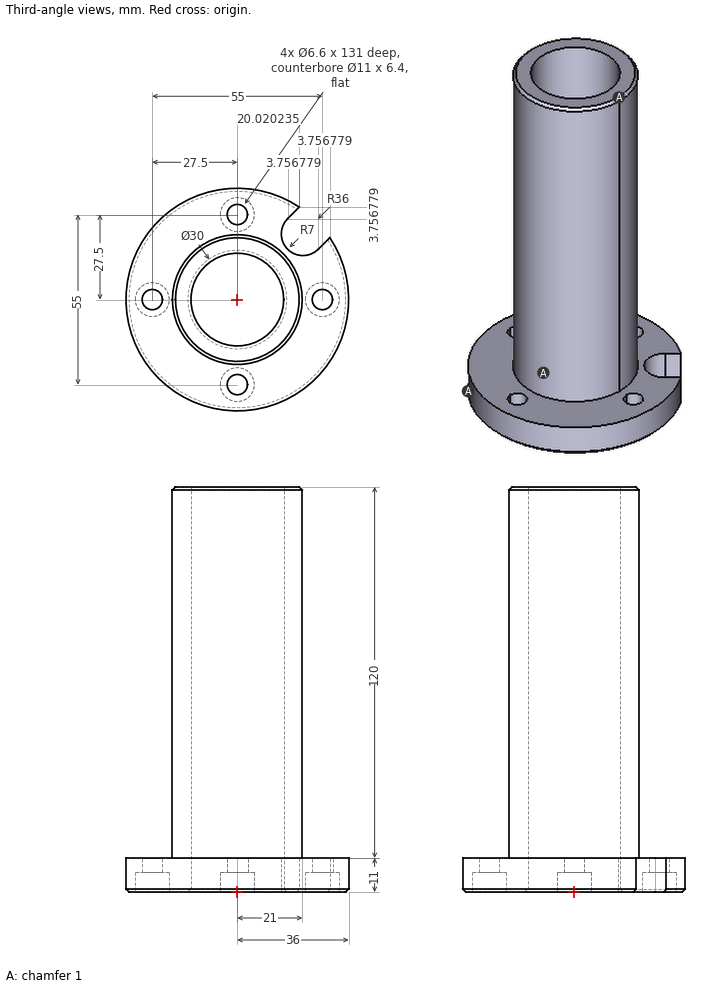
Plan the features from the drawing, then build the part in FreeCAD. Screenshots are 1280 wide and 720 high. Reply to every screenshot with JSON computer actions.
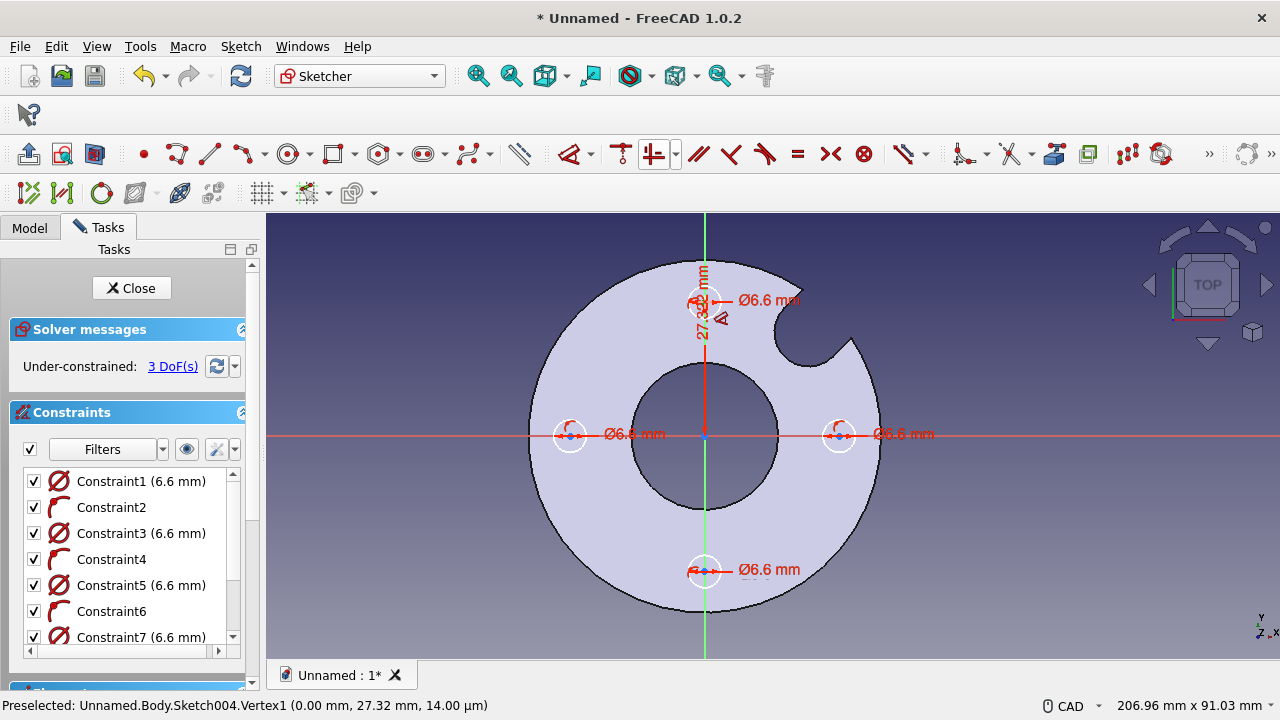
{"action": "left_click", "coordinate": [705, 572]}
{"action": "left_click", "coordinate": [739, 375]}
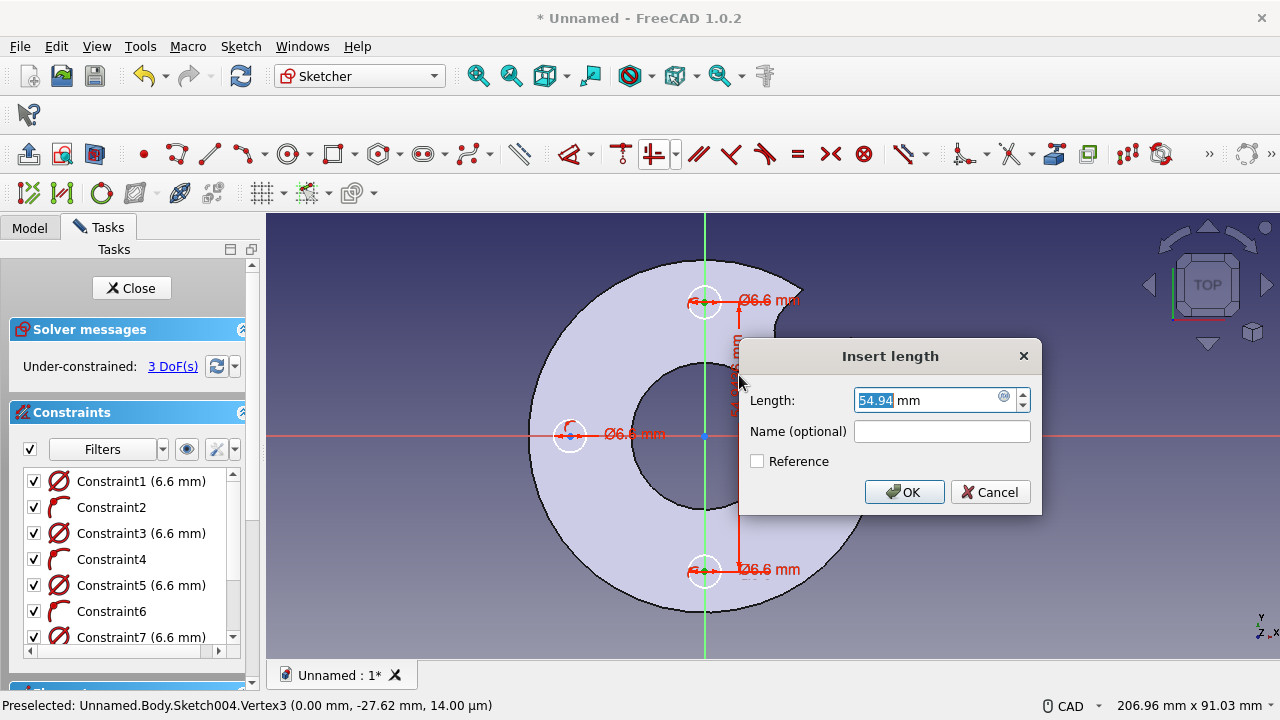
{"action": "type", "text": "55"}
{"action": "key", "text": "Return"}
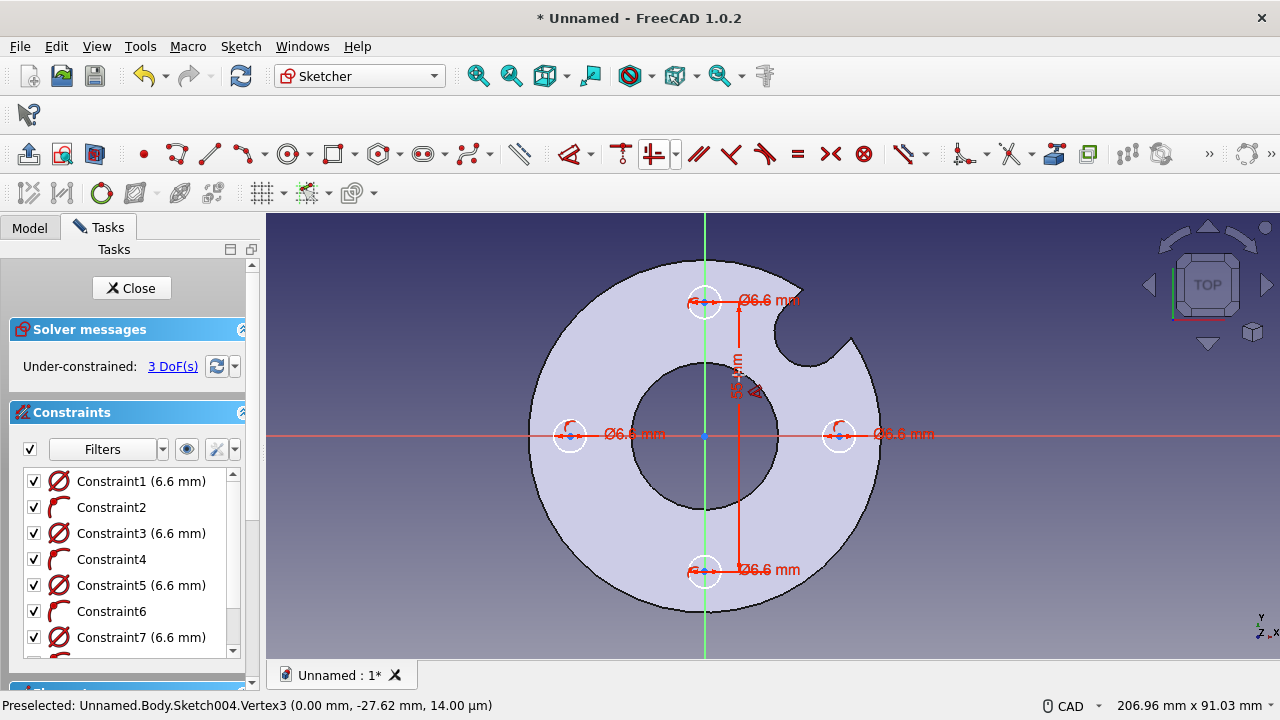
{"action": "left_click", "coordinate": [570, 436]}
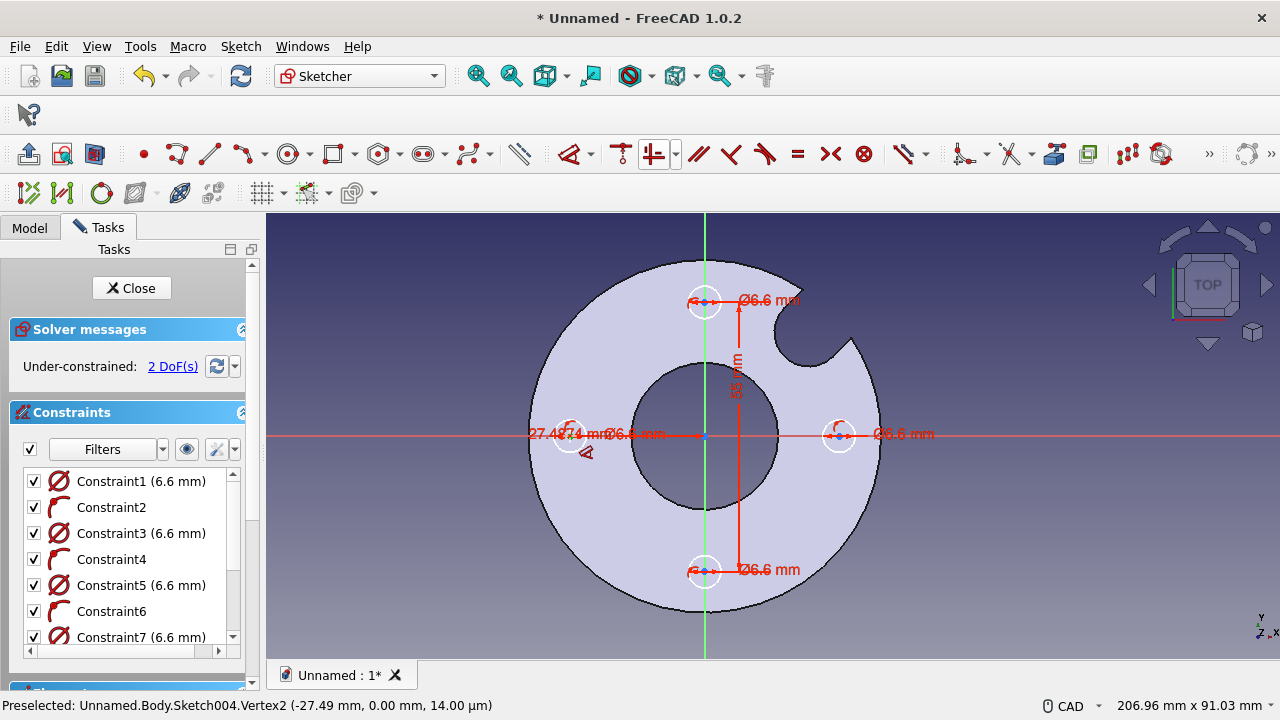
{"action": "left_click", "coordinate": [839, 436]}
{"action": "left_click", "coordinate": [643, 470]}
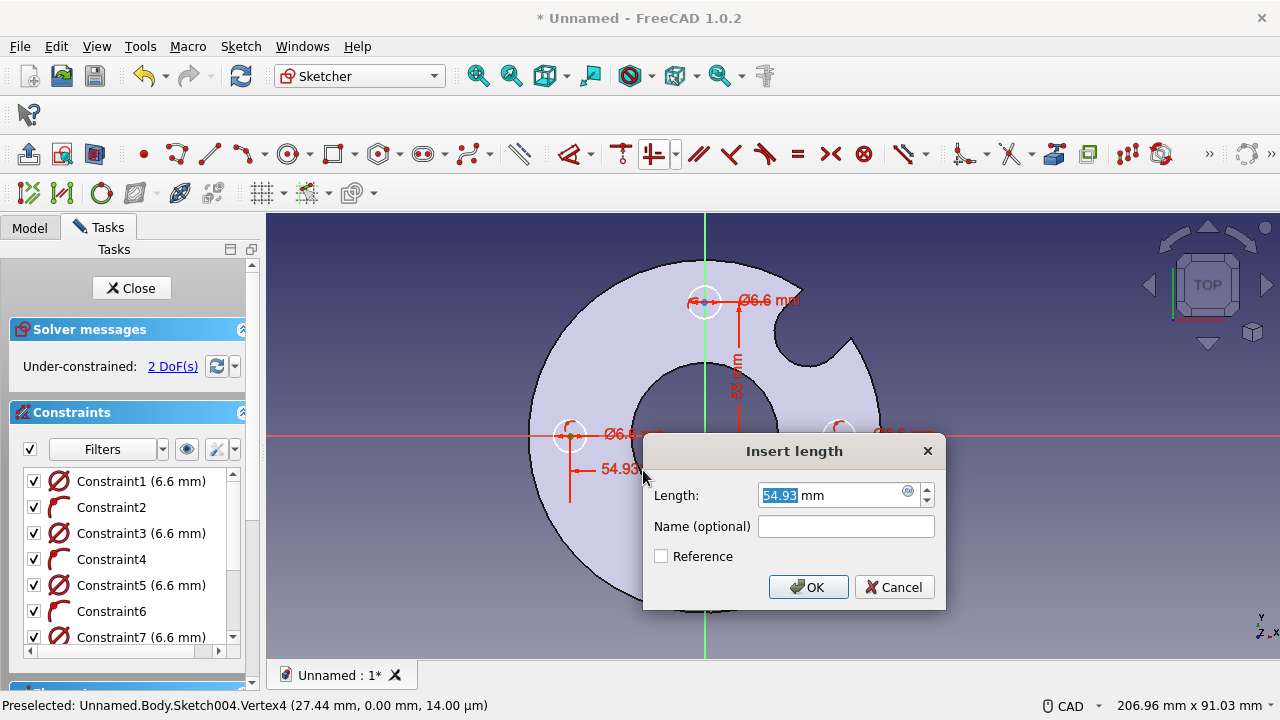
{"action": "type", "text": "55"}
{"action": "key", "text": "Return"}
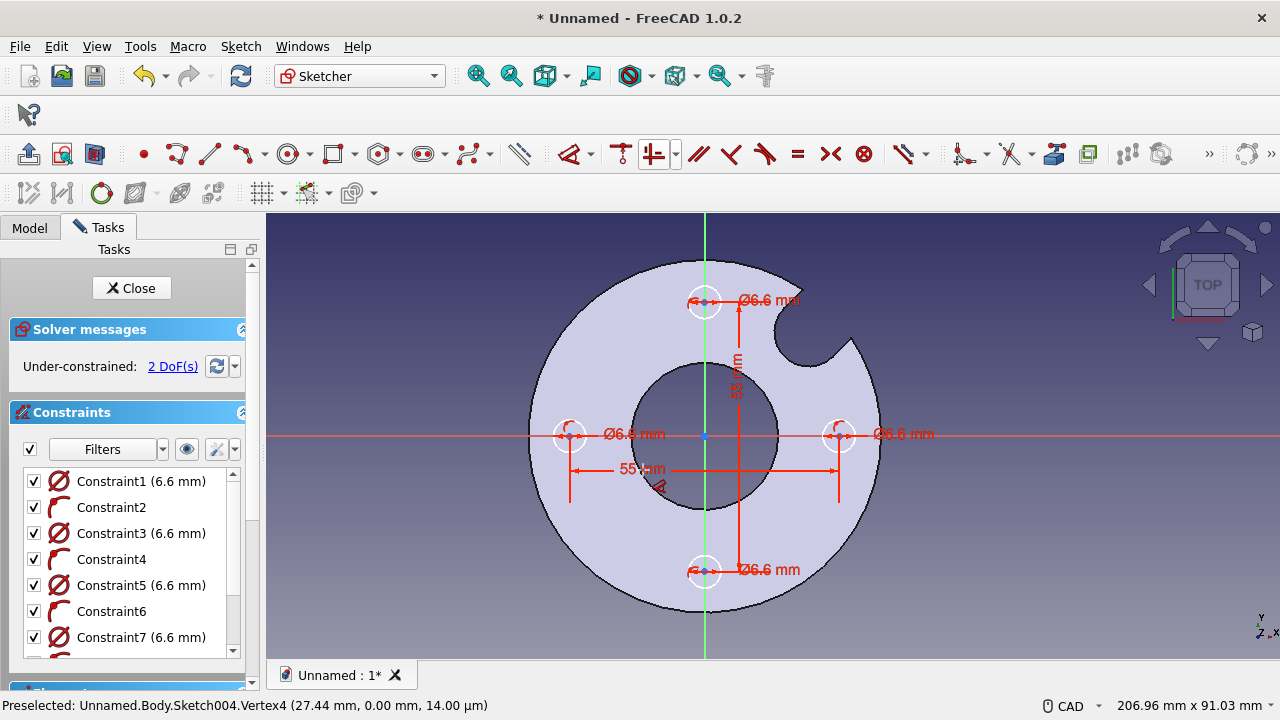
{"action": "left_click", "coordinate": [705, 302]}
{"action": "left_click", "coordinate": [739, 339]}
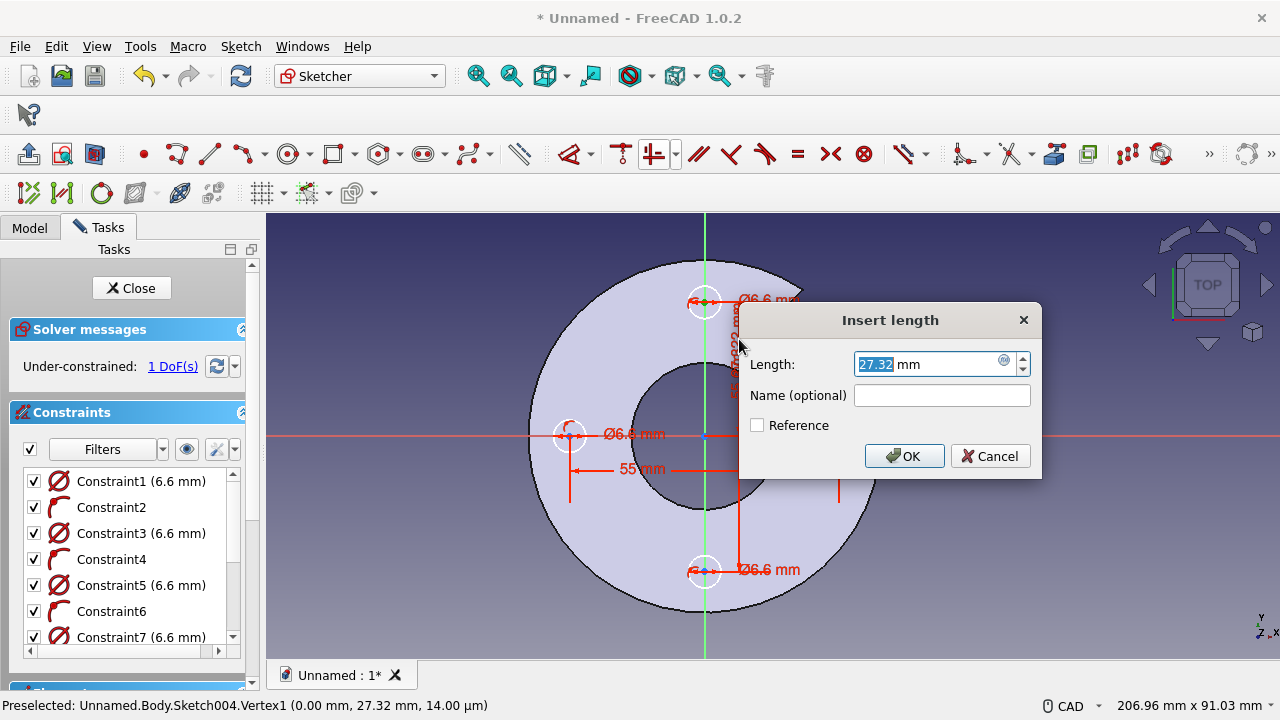
{"action": "type", "text": "27.5"}
{"action": "key", "text": "Return"}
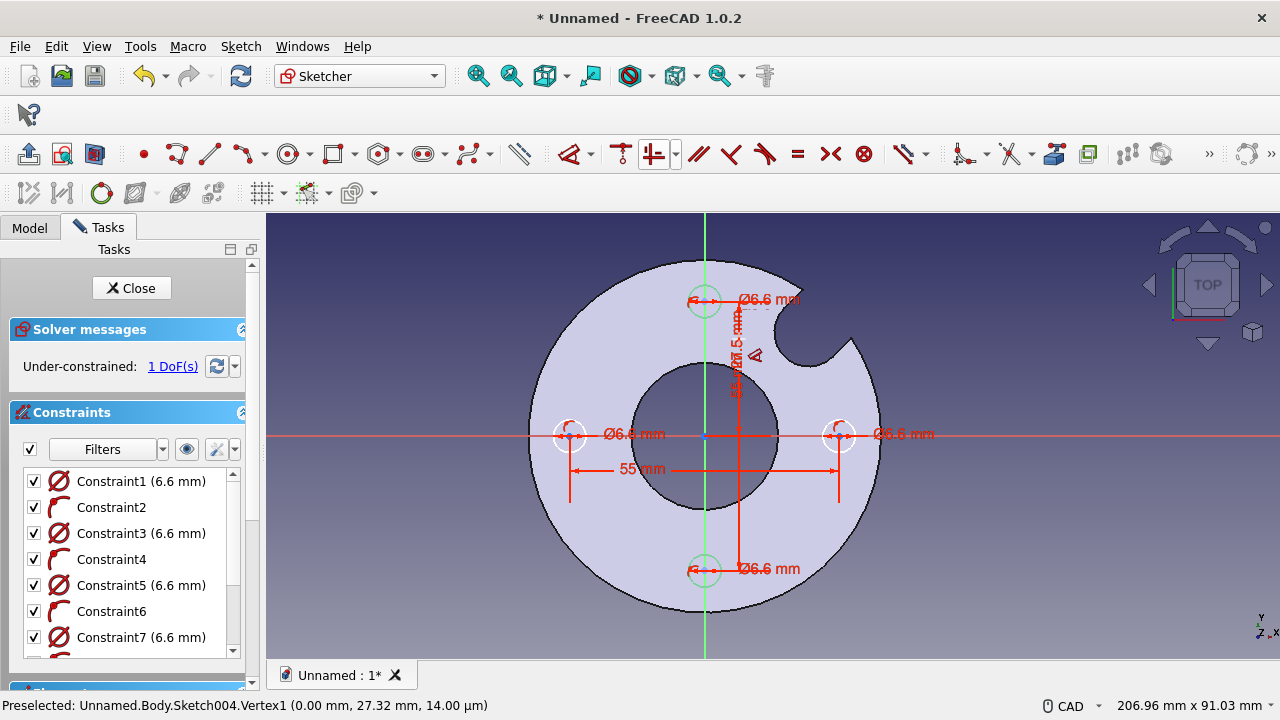
{"action": "left_click", "coordinate": [570, 436]}
{"action": "left_click", "coordinate": [637, 402]}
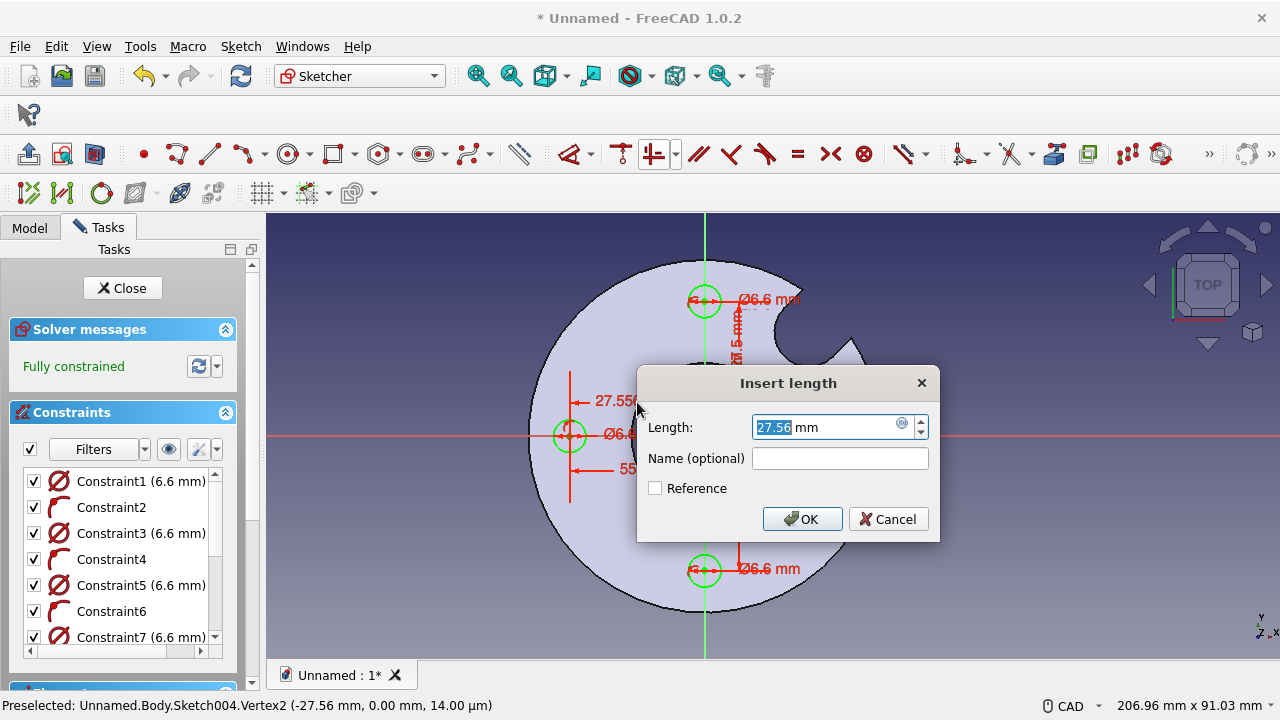
{"action": "type", "text": "27.5"}
{"action": "key", "text": "Return"}
{"action": "key", "text": "Escape"}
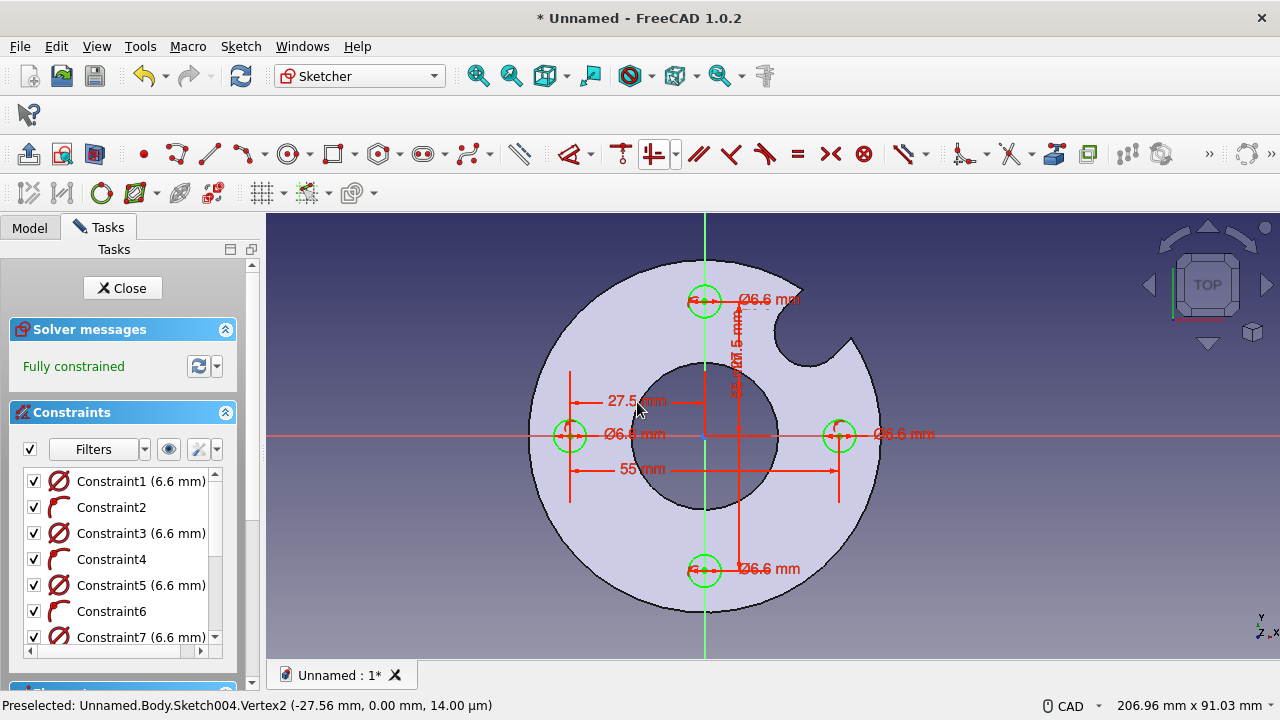
{"action": "left_click", "coordinate": [123, 288]}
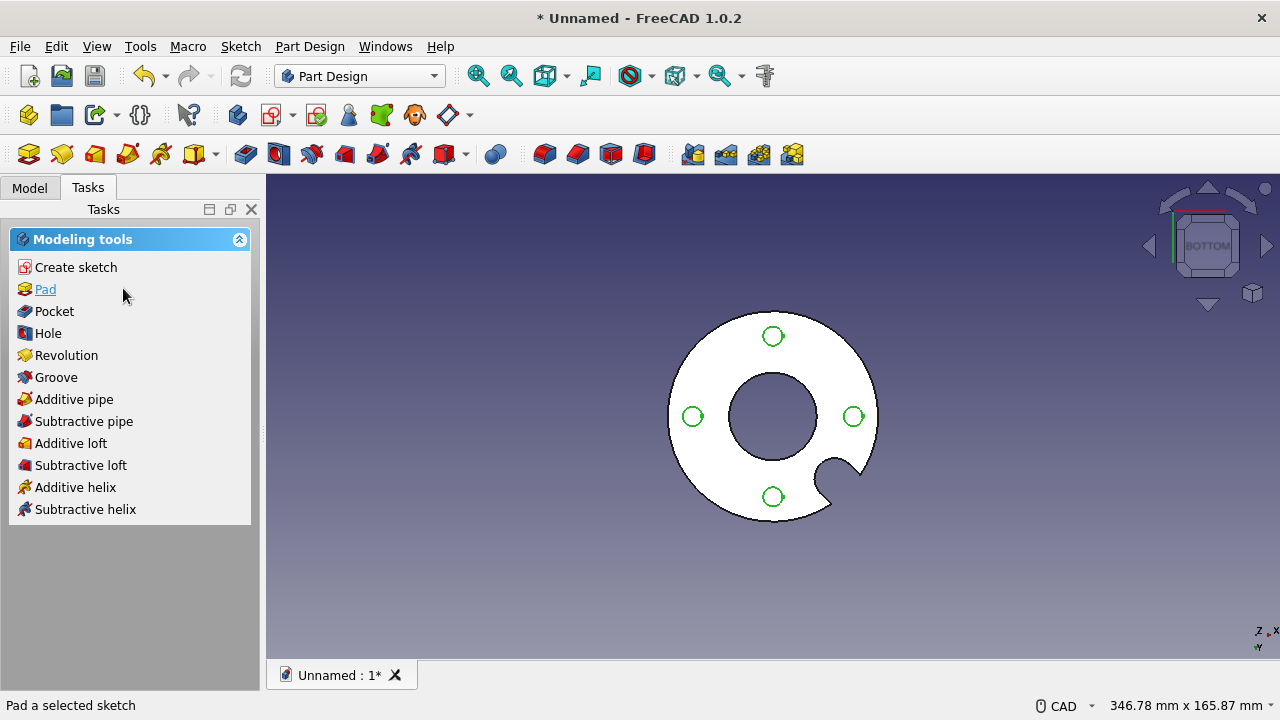
{"action": "left_click", "coordinate": [279, 154]}